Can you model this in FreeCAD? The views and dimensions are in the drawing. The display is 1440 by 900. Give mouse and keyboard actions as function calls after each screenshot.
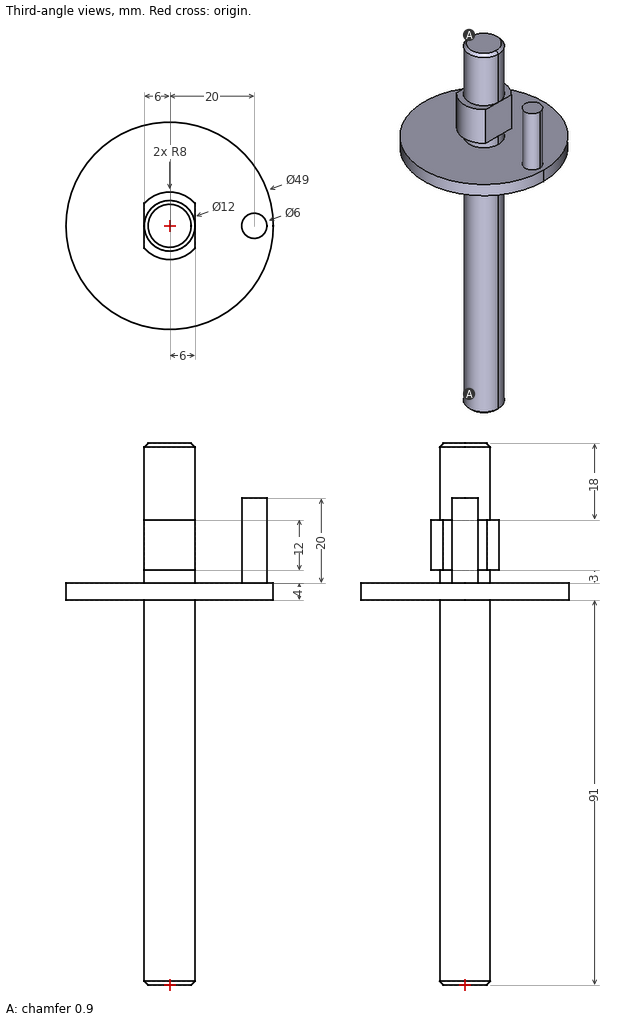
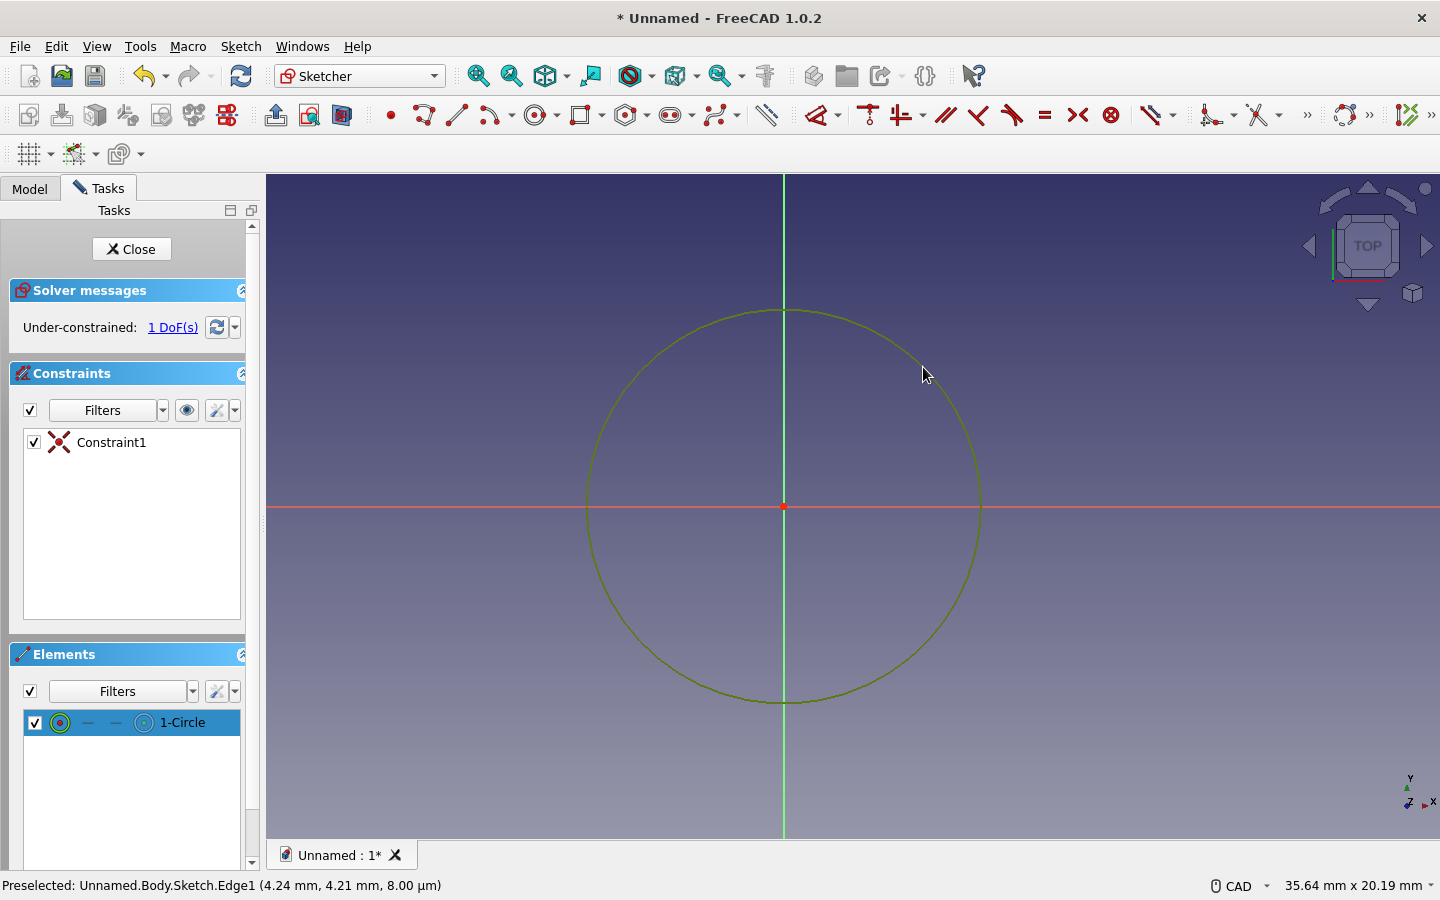
key(k)
key(o)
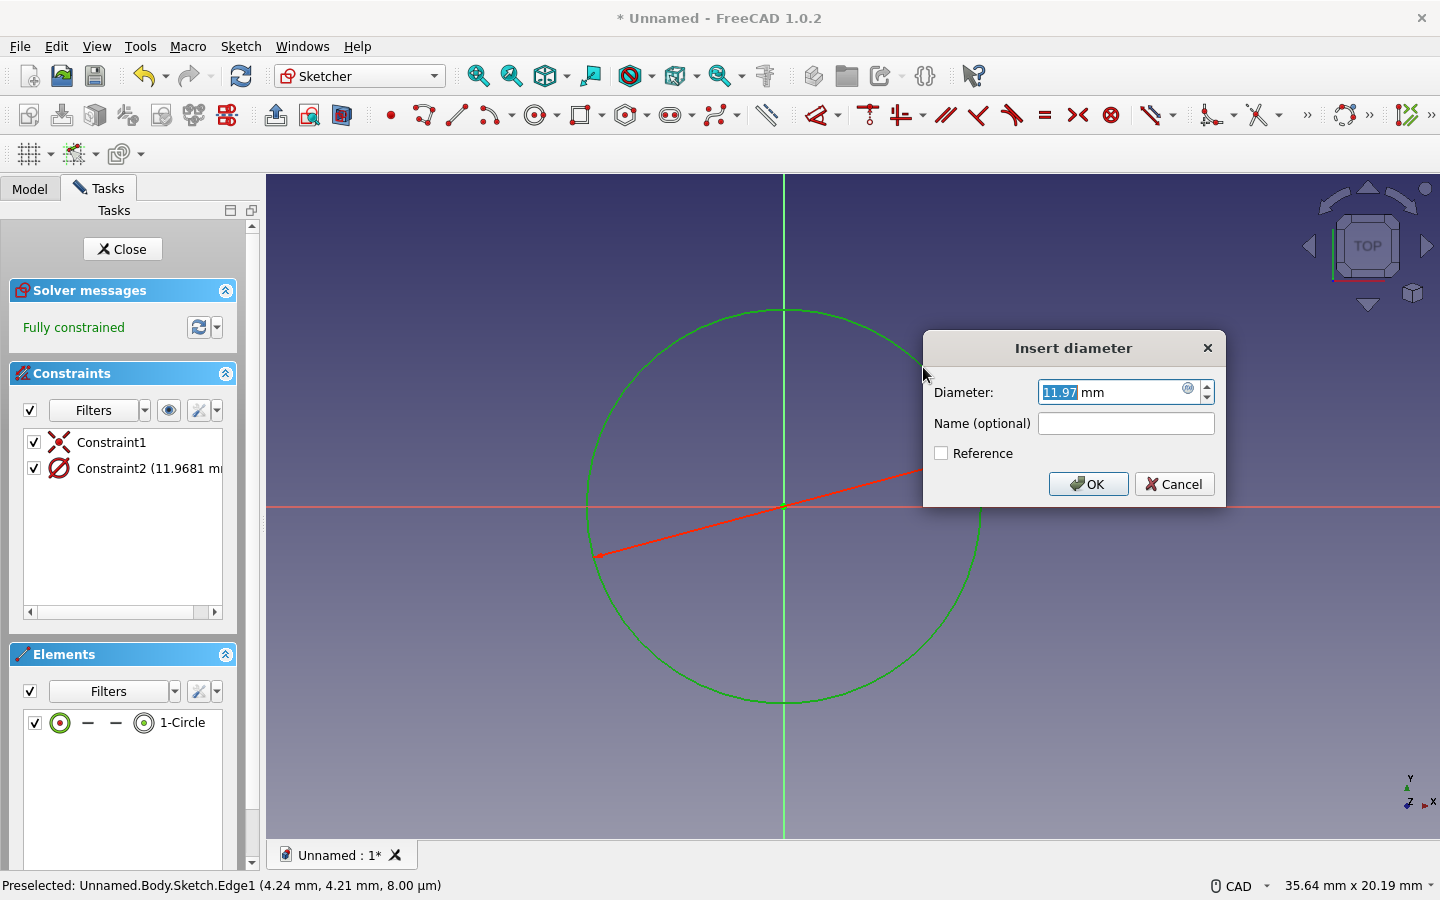
text(12)
key(Return)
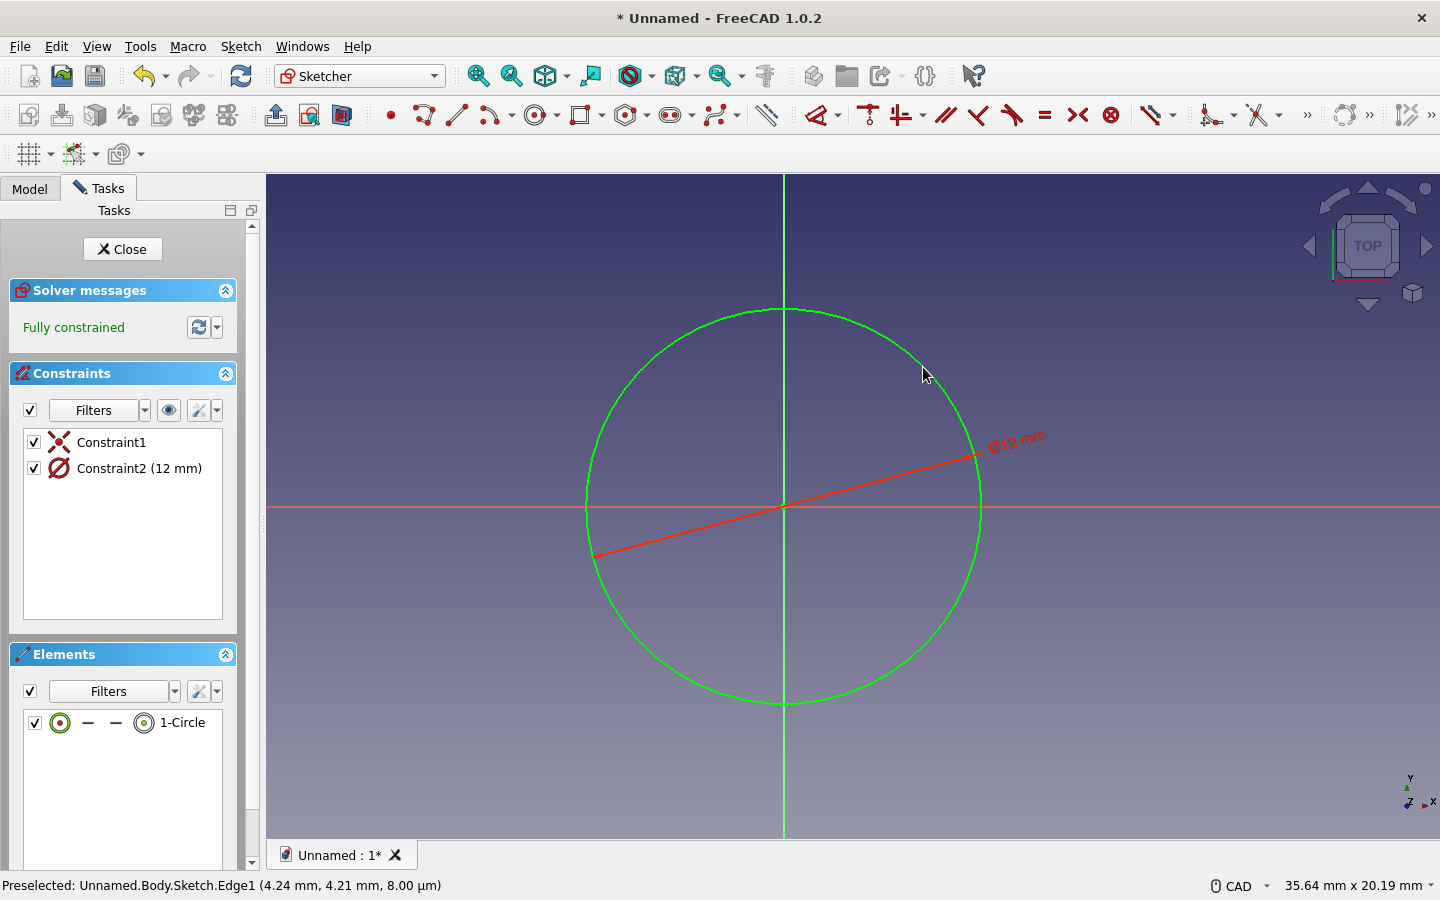
click(123, 249)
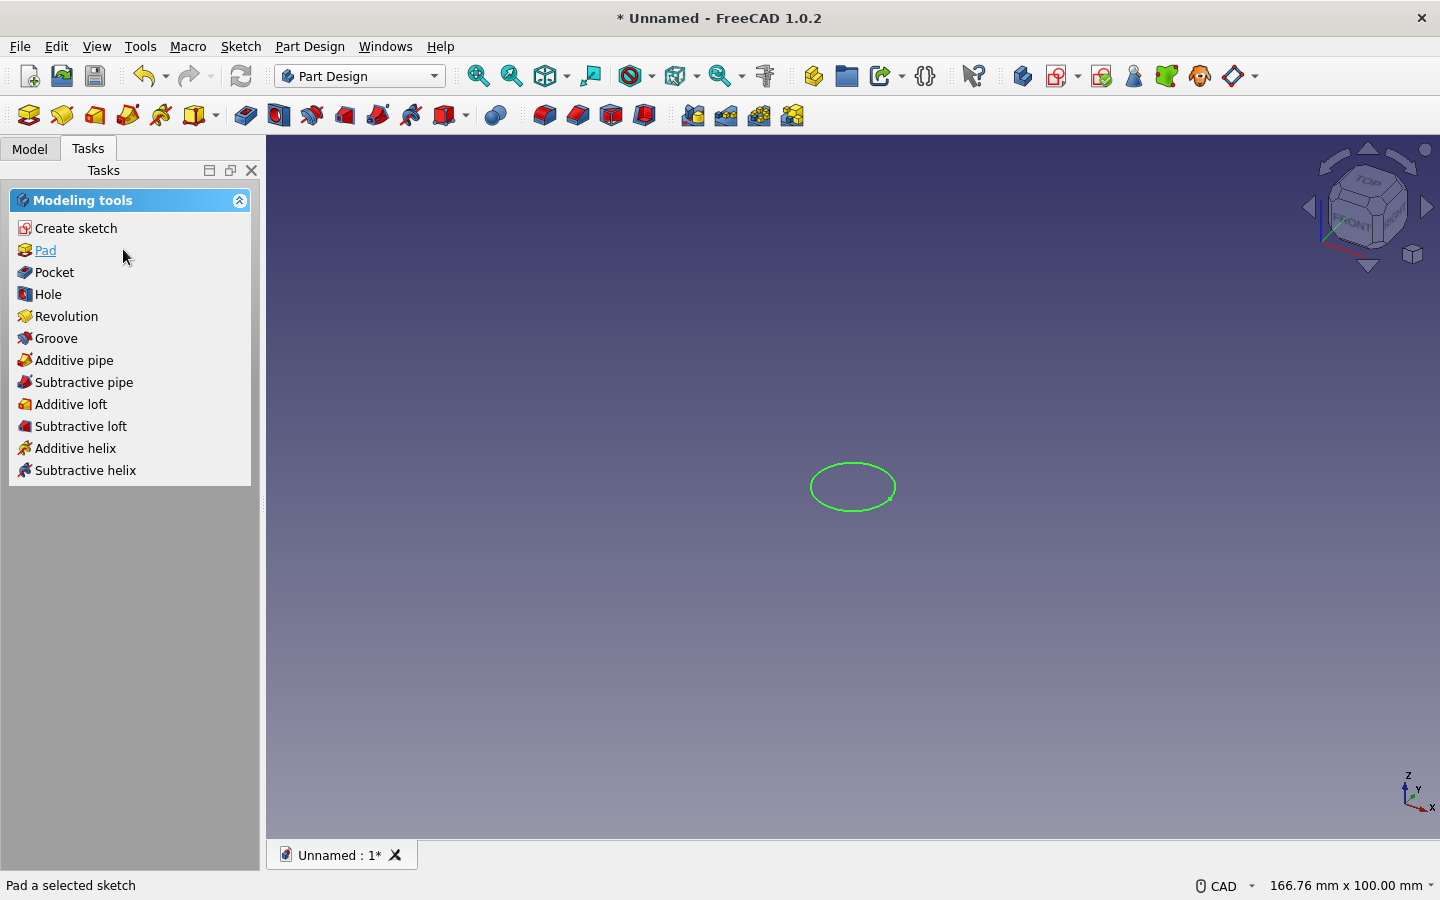
click(29, 116)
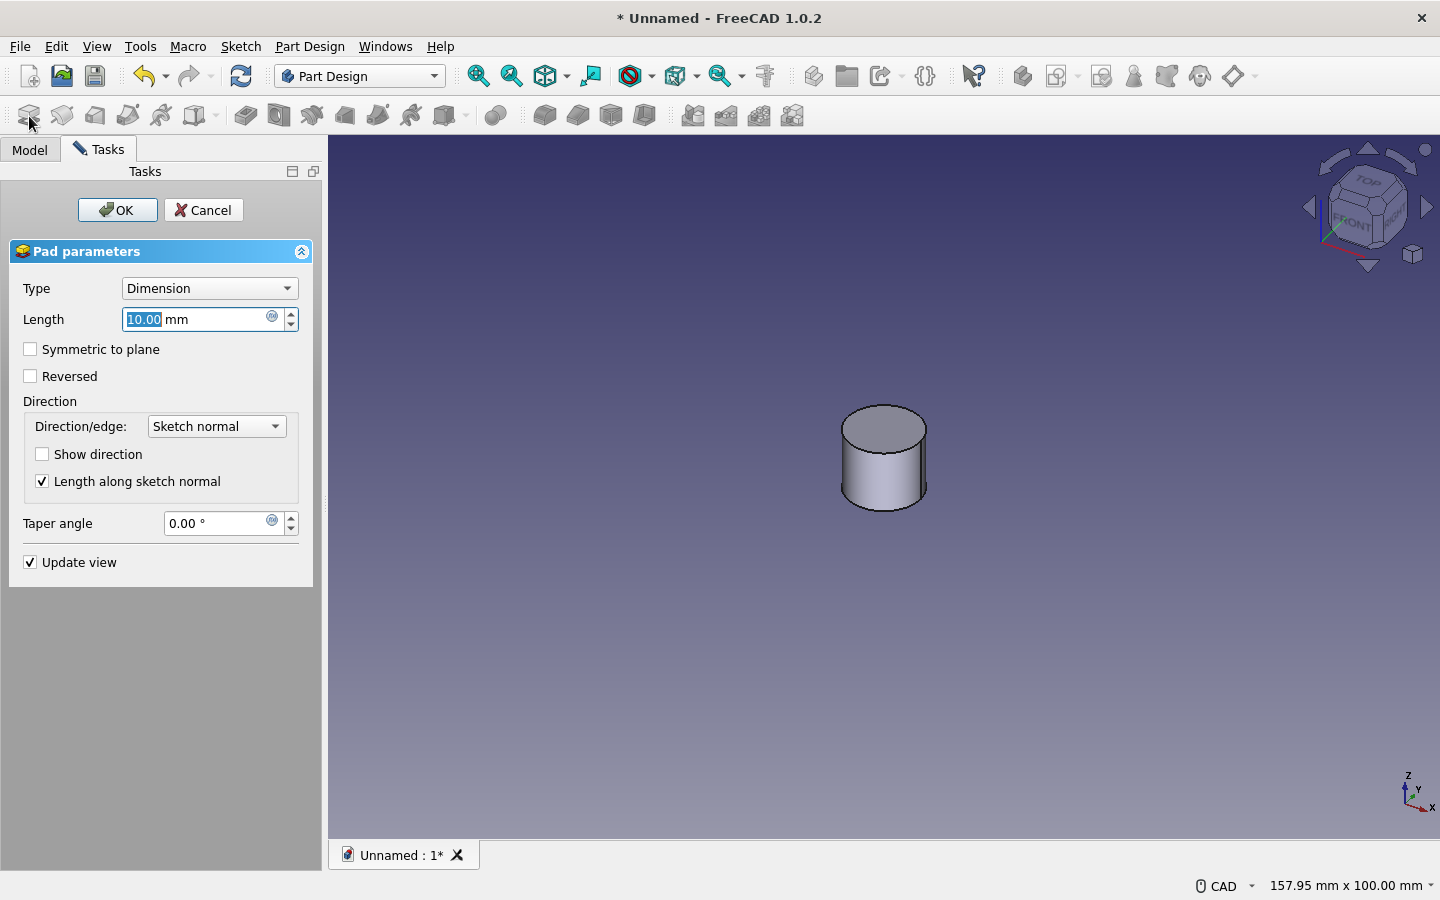
text(91)
key(Tab)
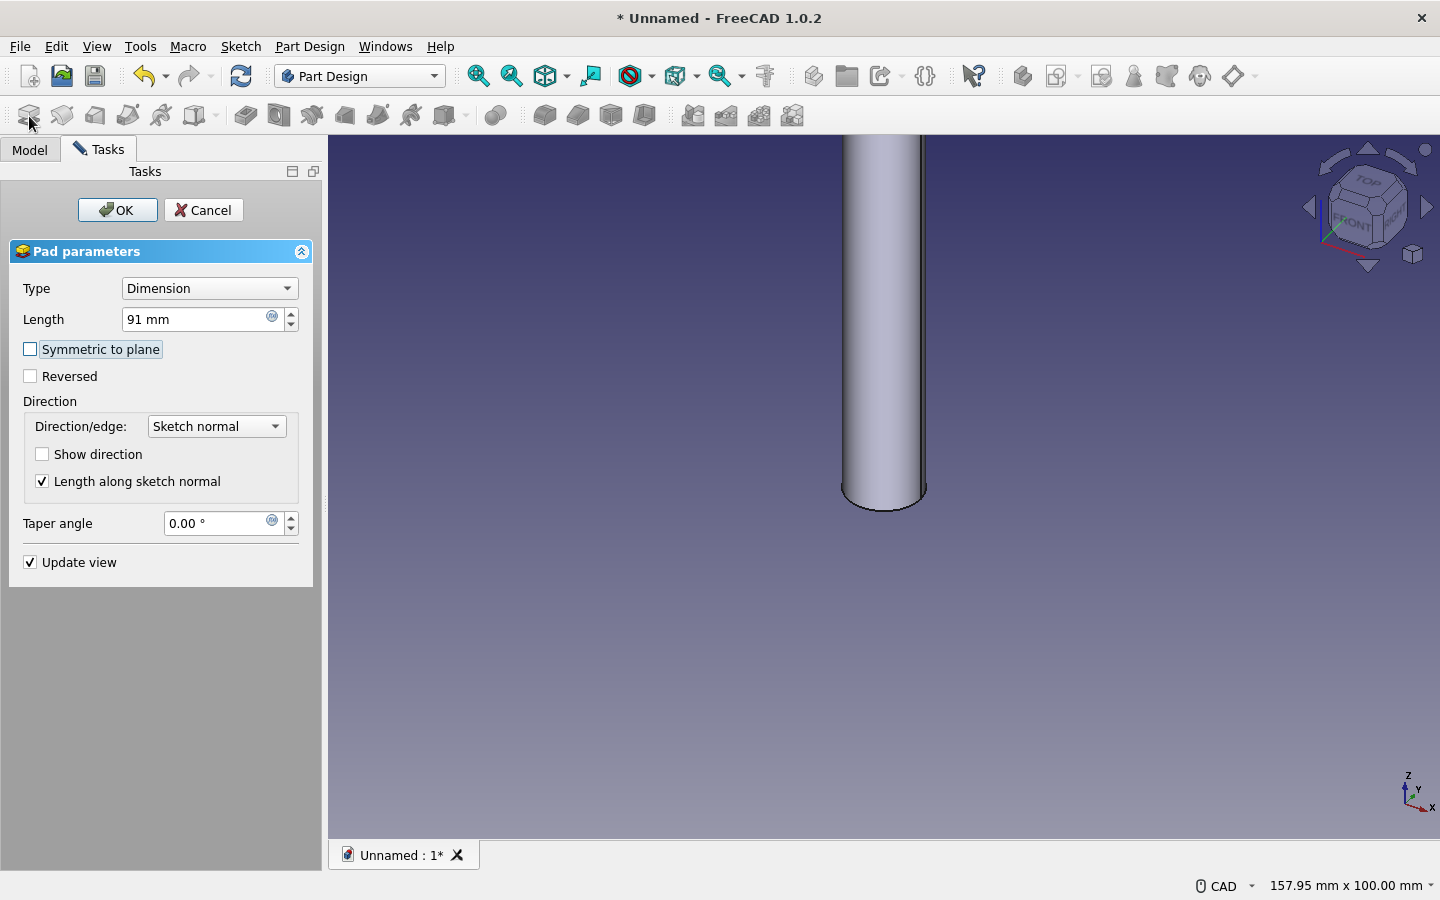
click(118, 210)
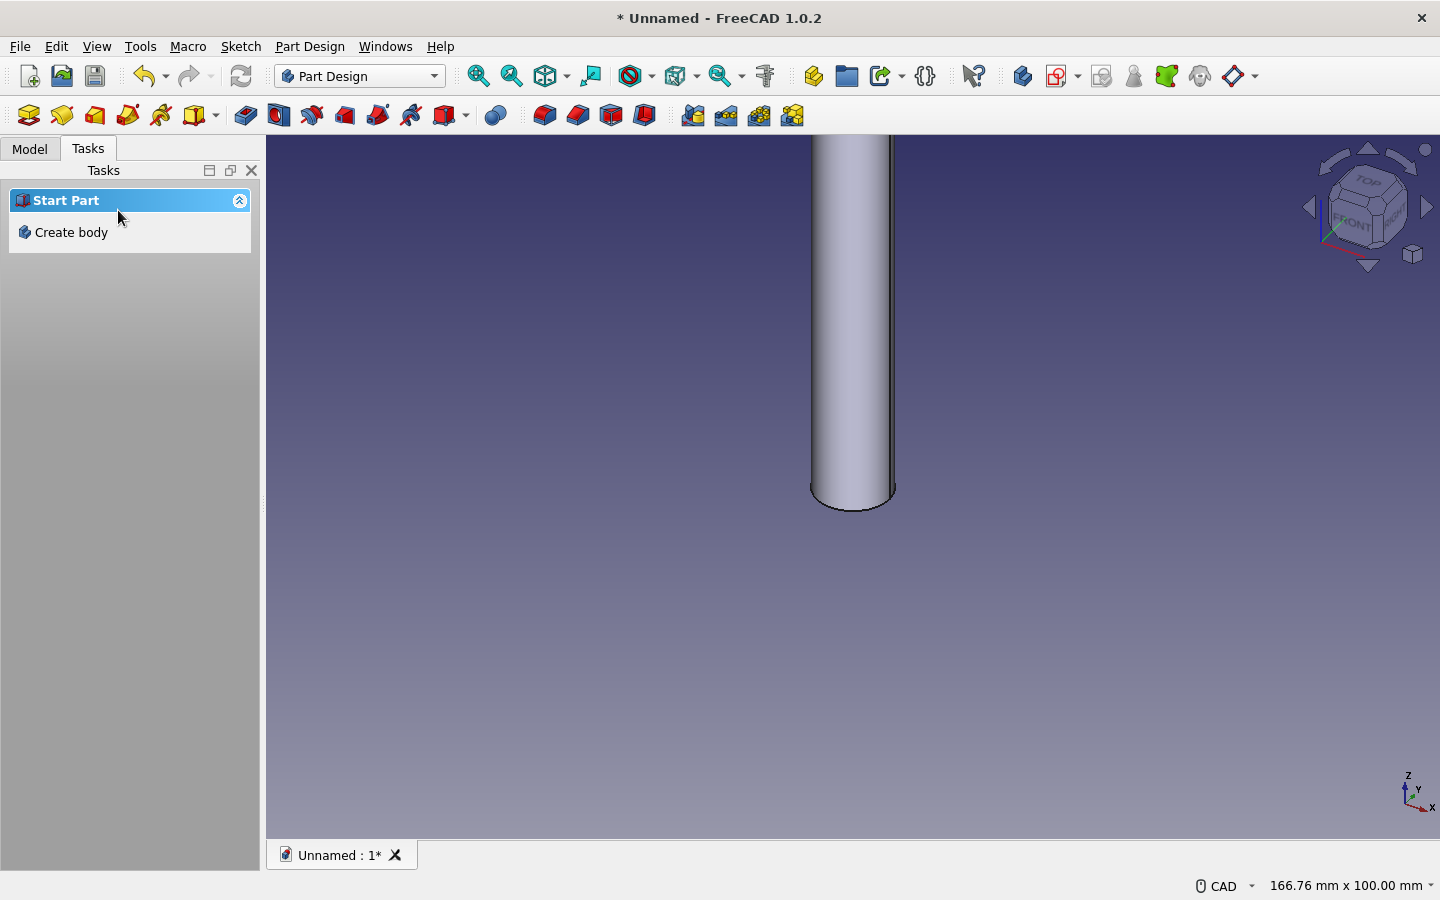
click(479, 76)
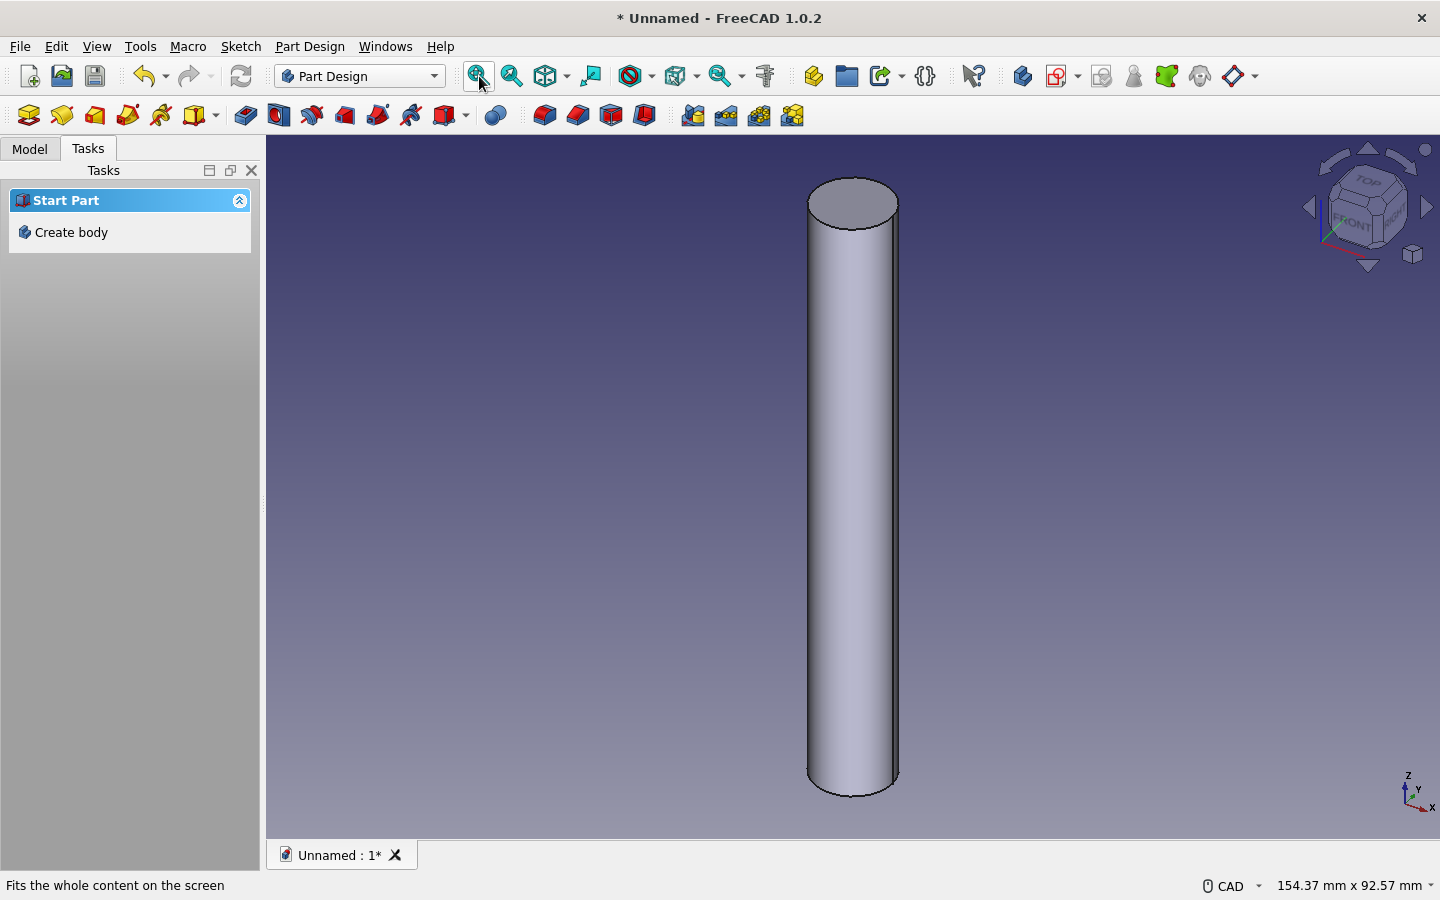
click(853, 203)